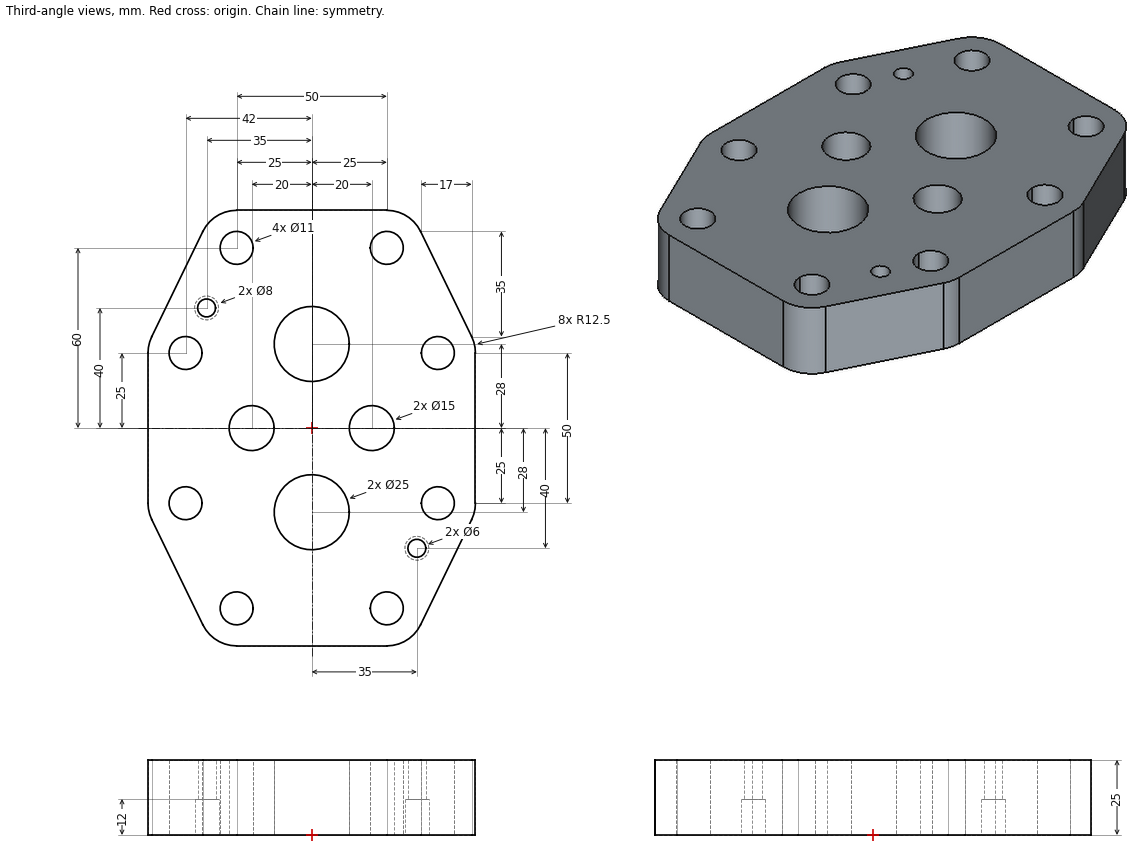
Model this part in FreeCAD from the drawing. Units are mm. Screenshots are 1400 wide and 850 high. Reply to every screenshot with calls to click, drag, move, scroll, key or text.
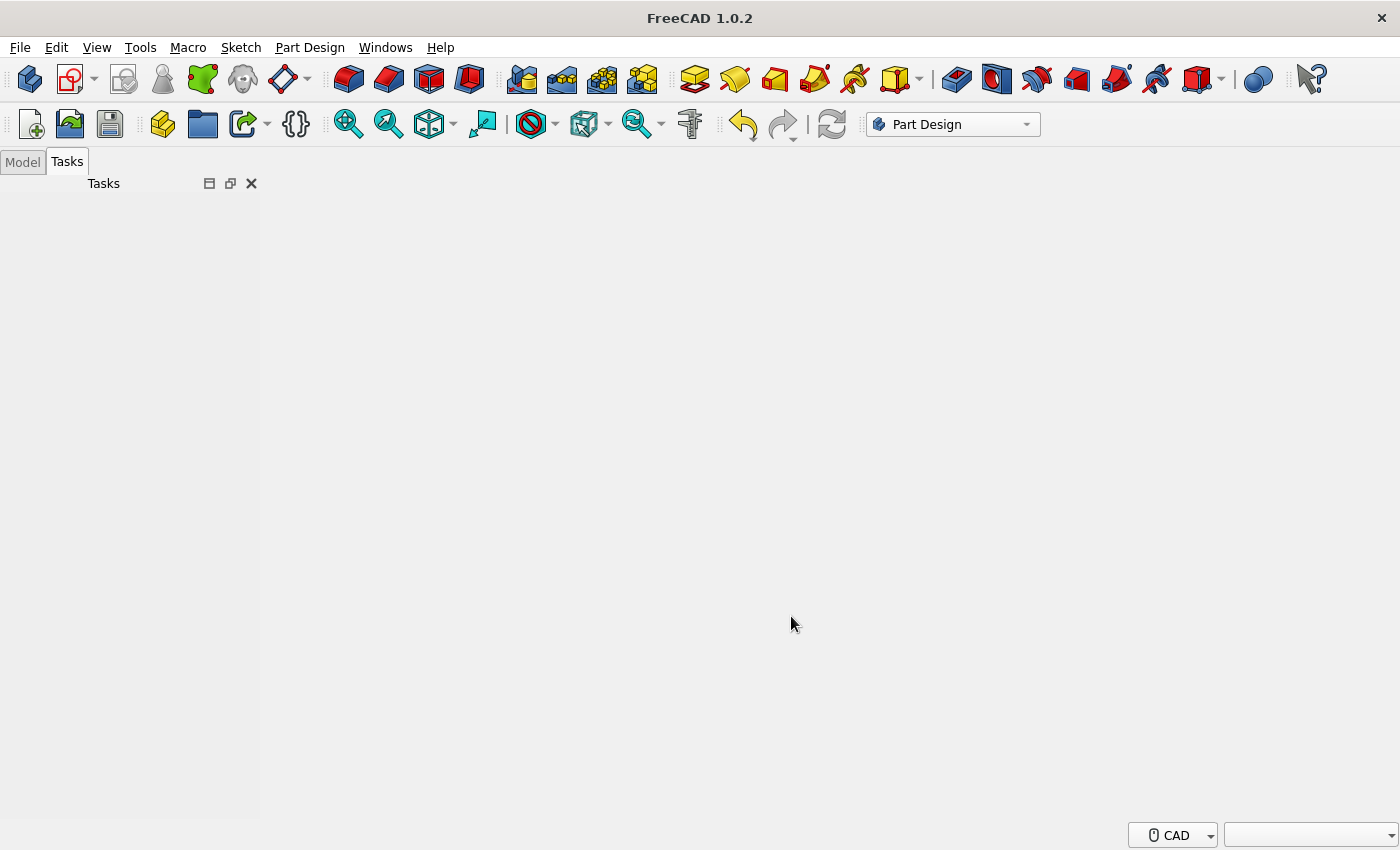
key(ctrl+n)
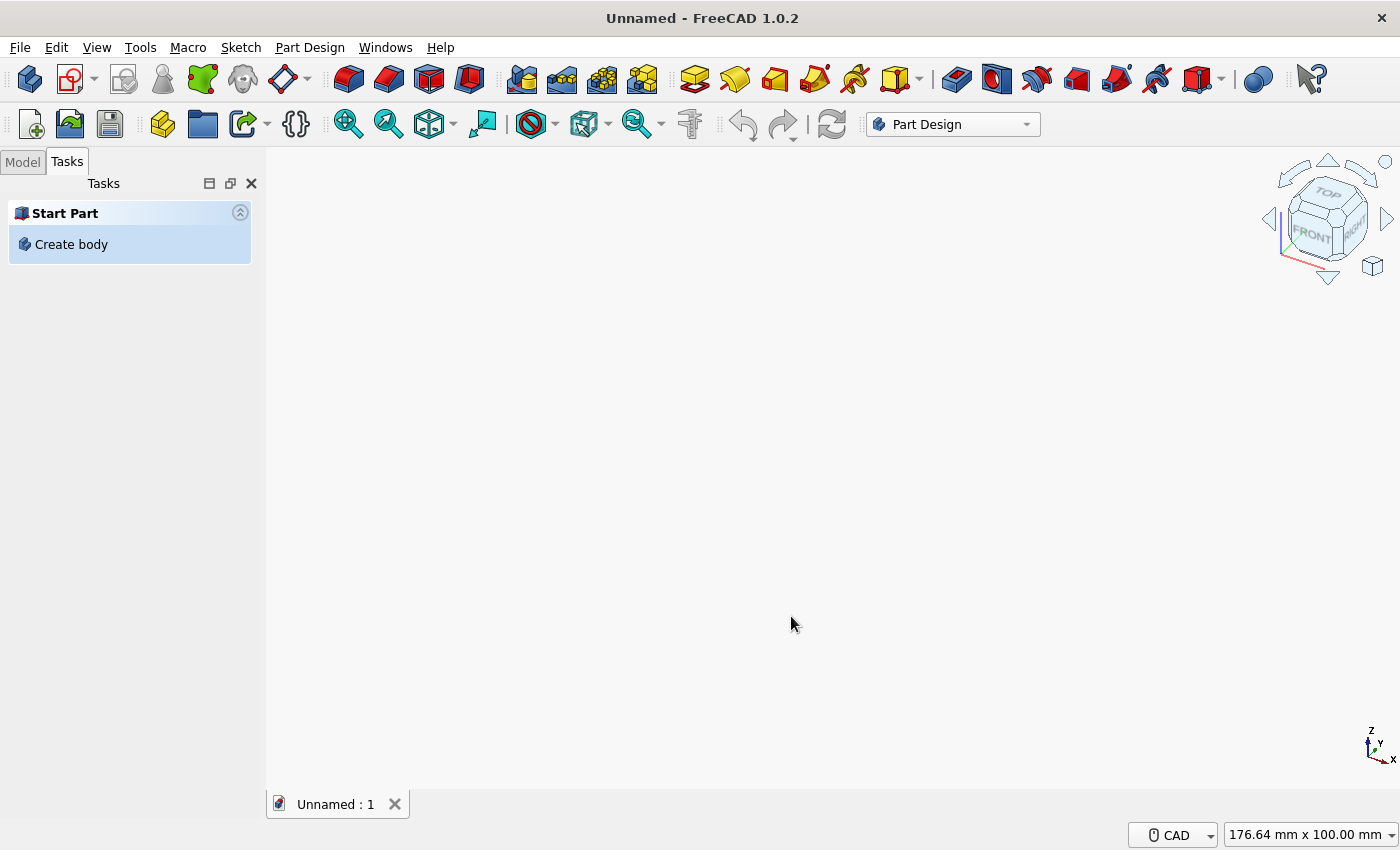
click(70, 80)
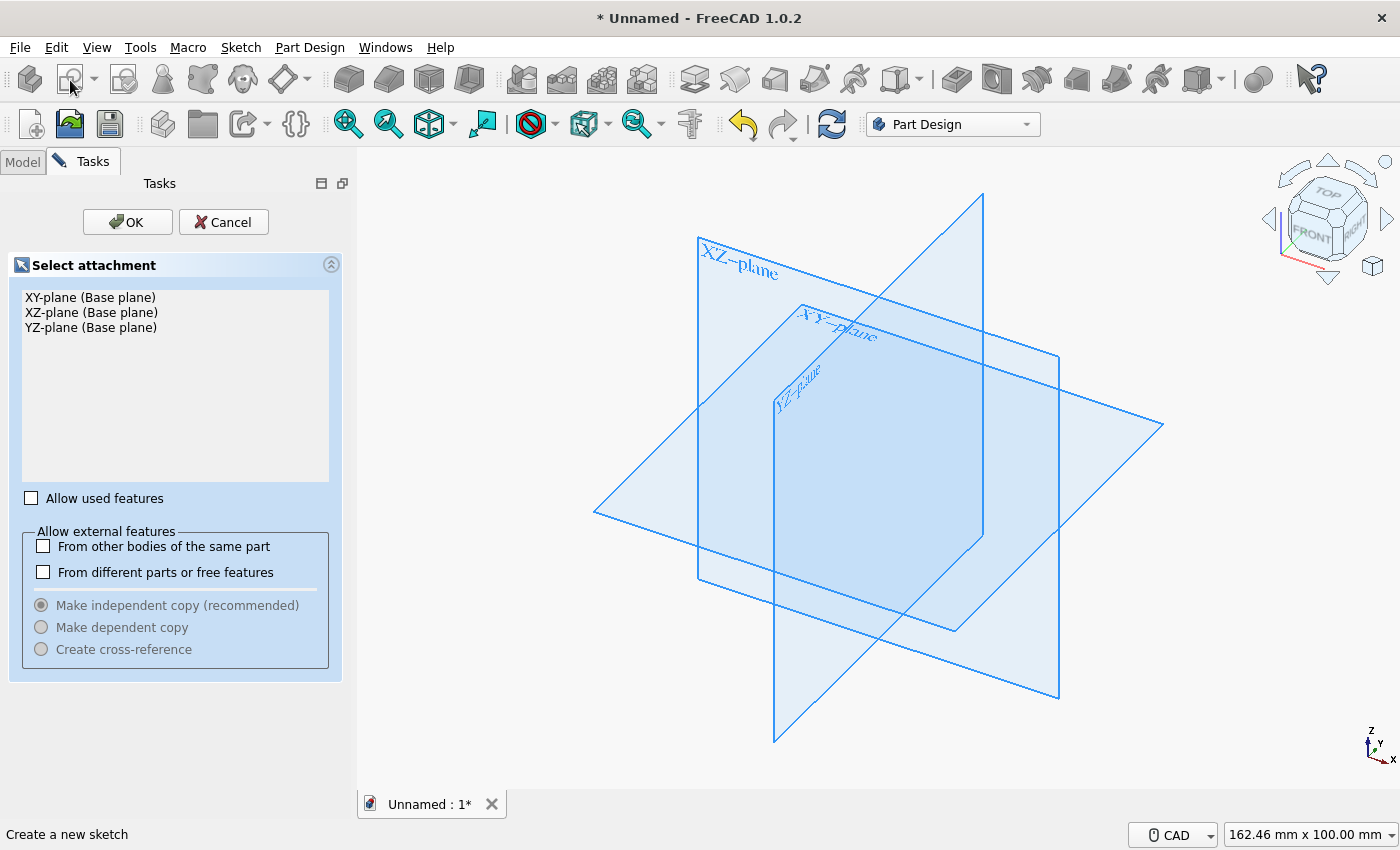
click(82, 298)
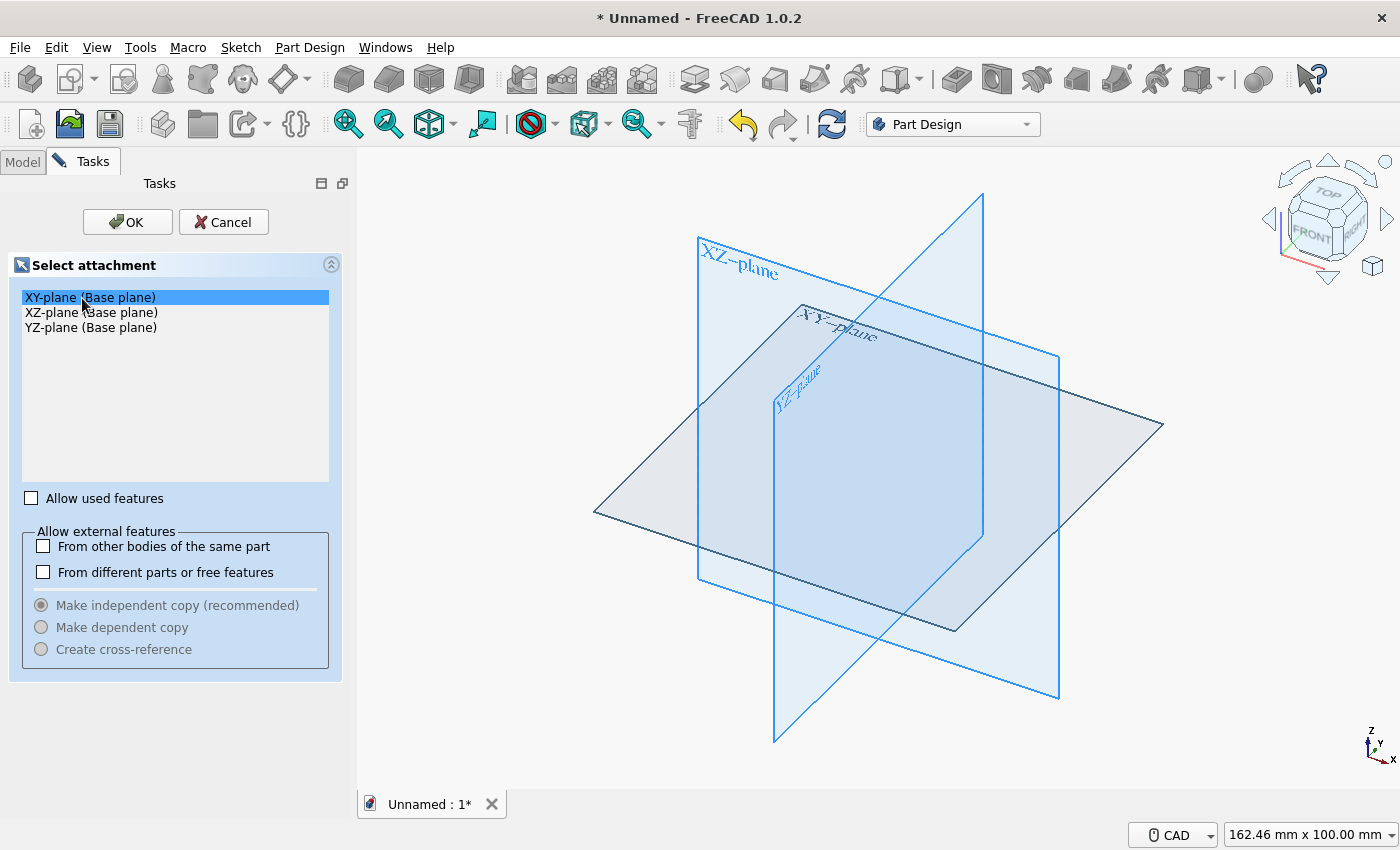
click(128, 222)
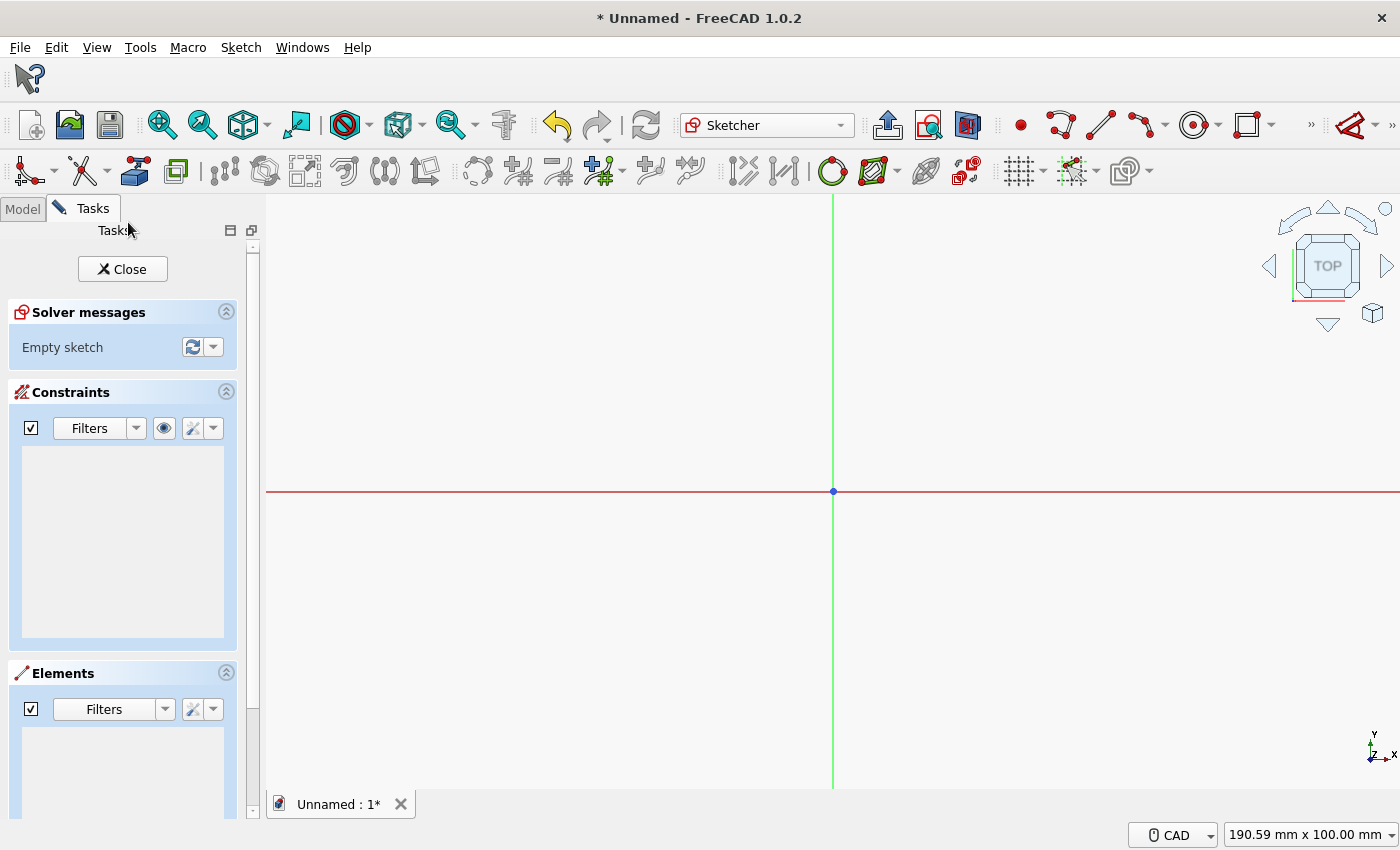
scroll(709, 492, down, 4)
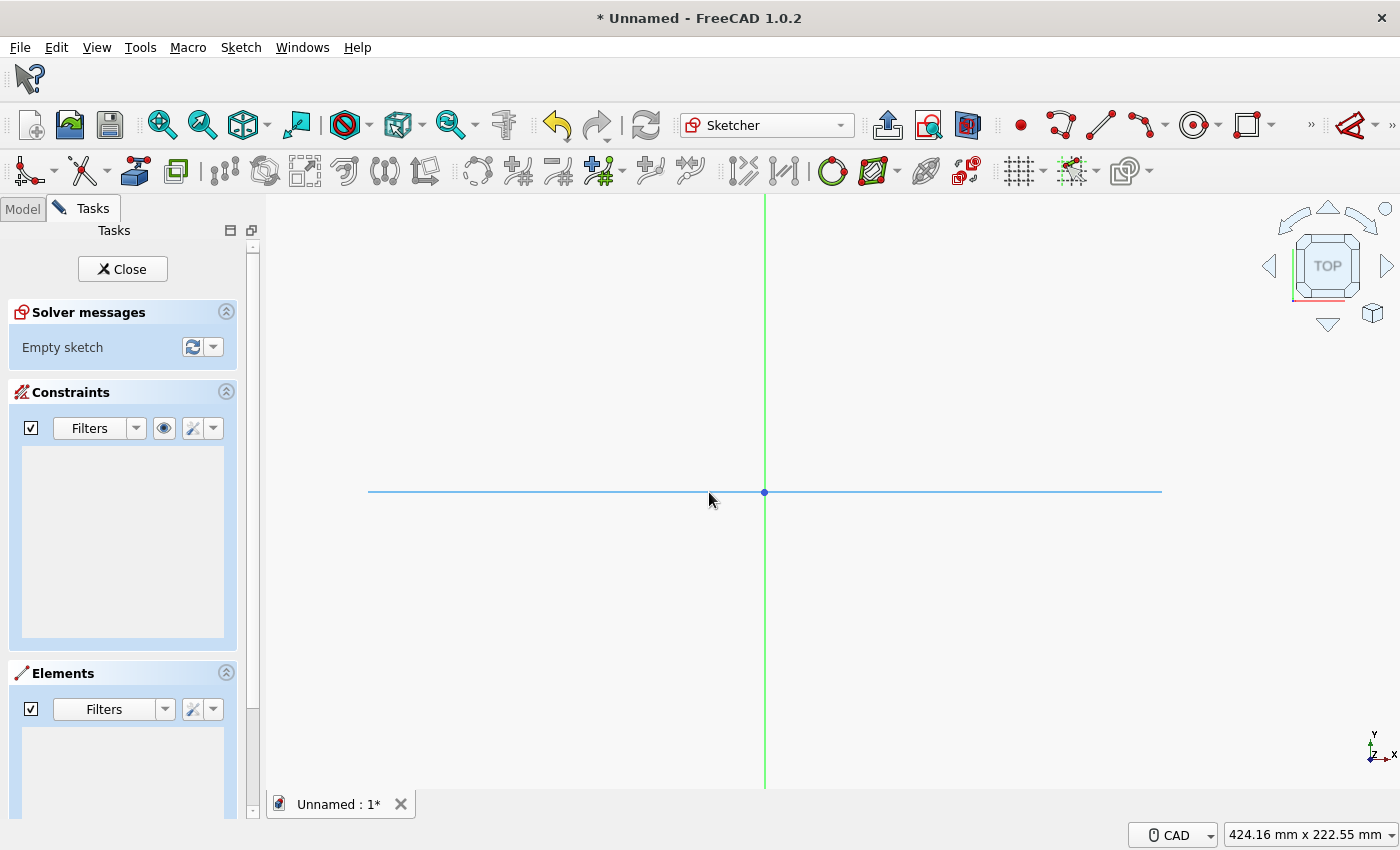
key(g)
key(l)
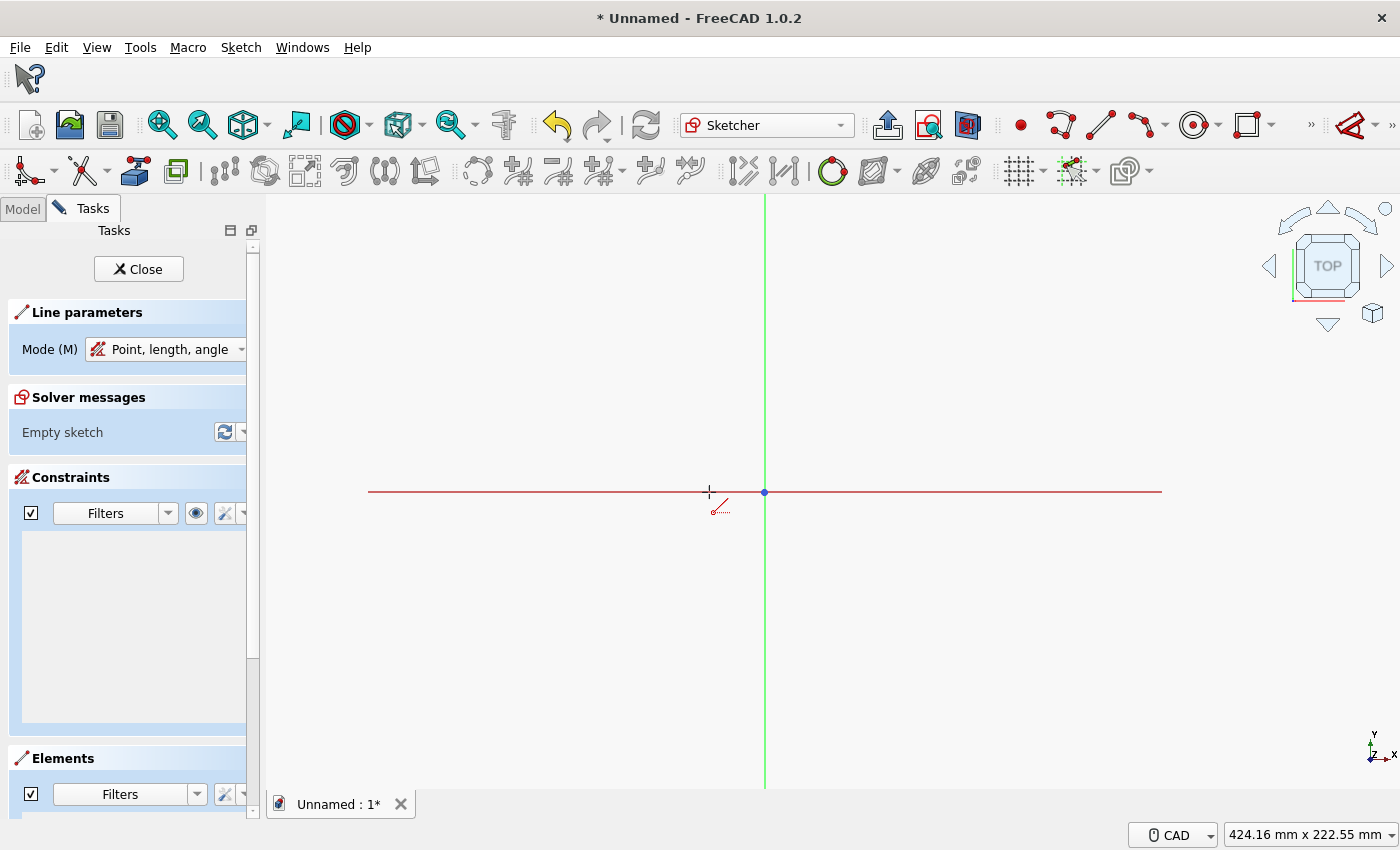
click(911, 559)
click(911, 425)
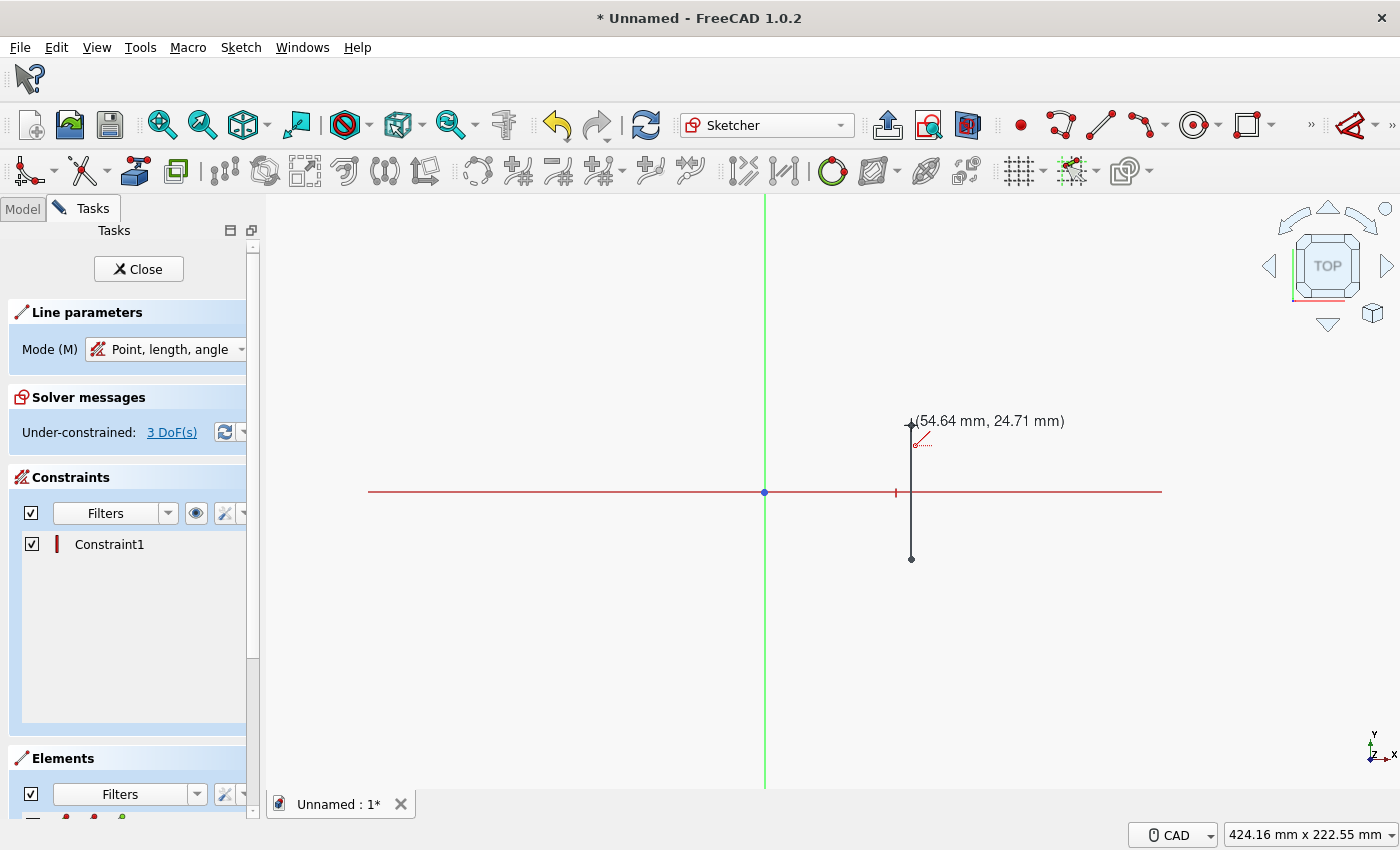
click(907, 411)
click(862, 317)